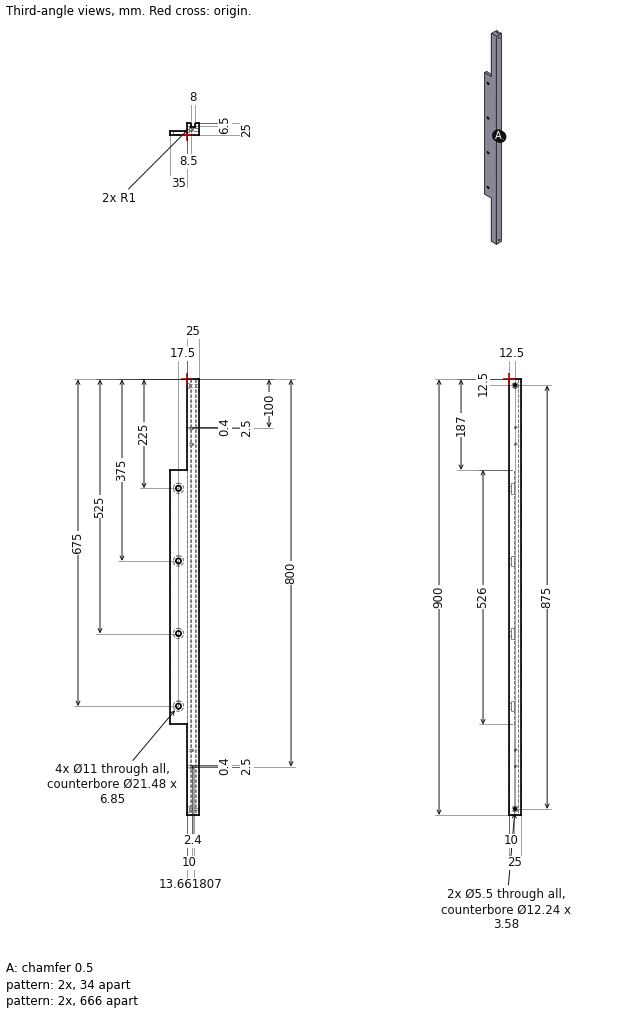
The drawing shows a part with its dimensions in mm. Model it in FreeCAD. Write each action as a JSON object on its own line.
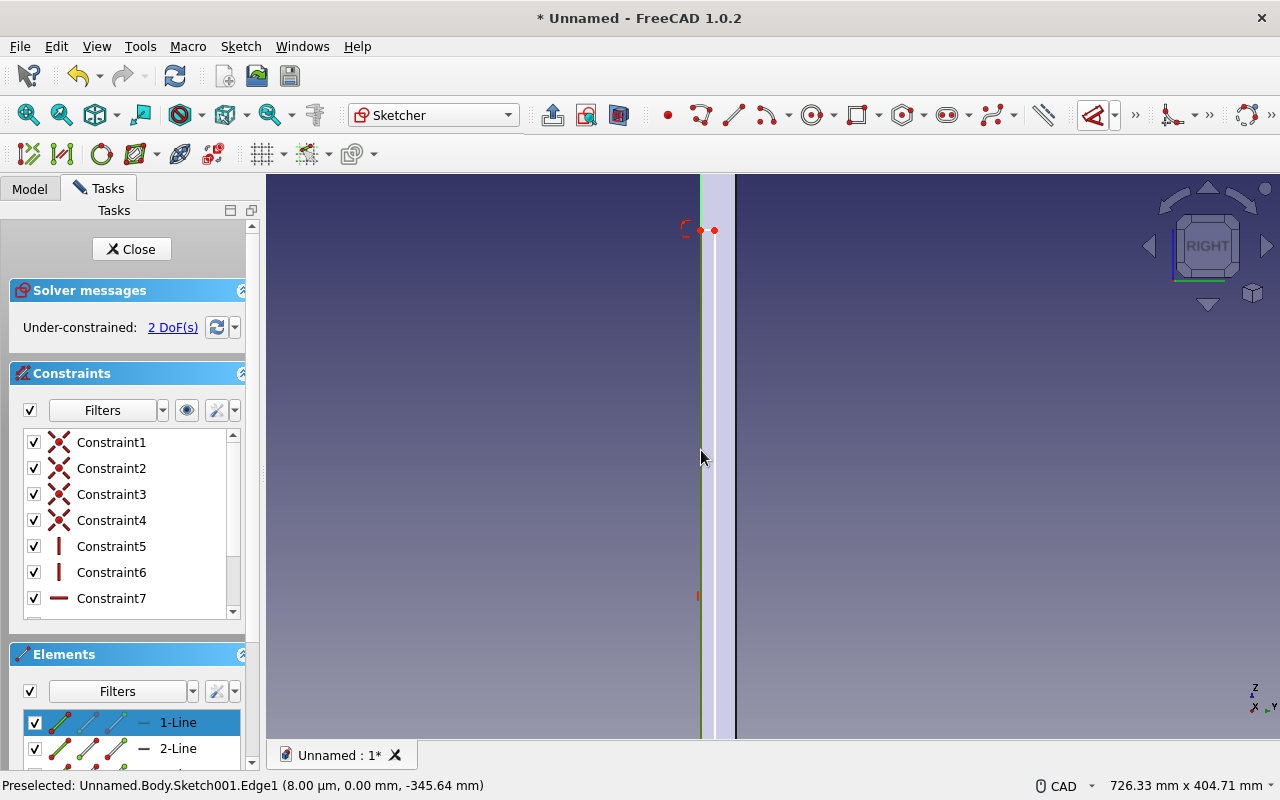
{"action": "key", "text": "i"}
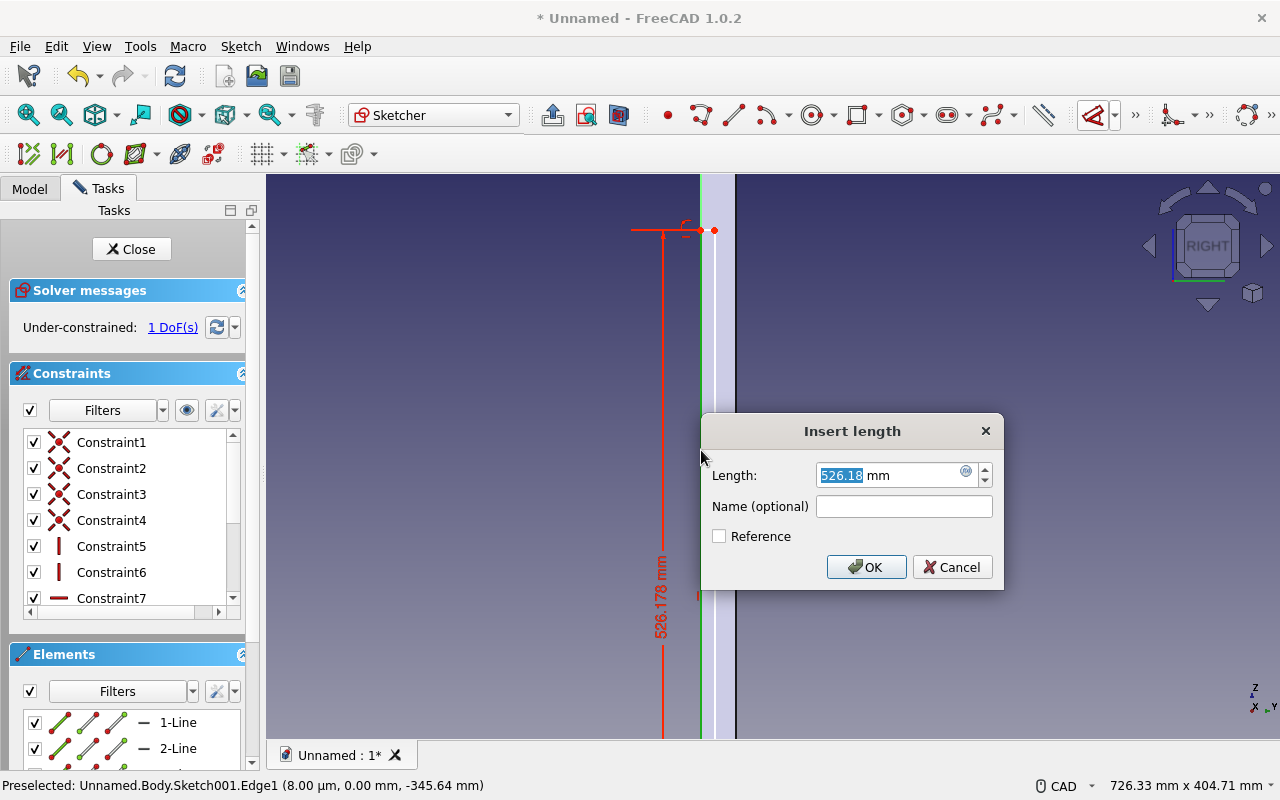
{"action": "type", "text": "526"}
{"action": "key", "text": "Return"}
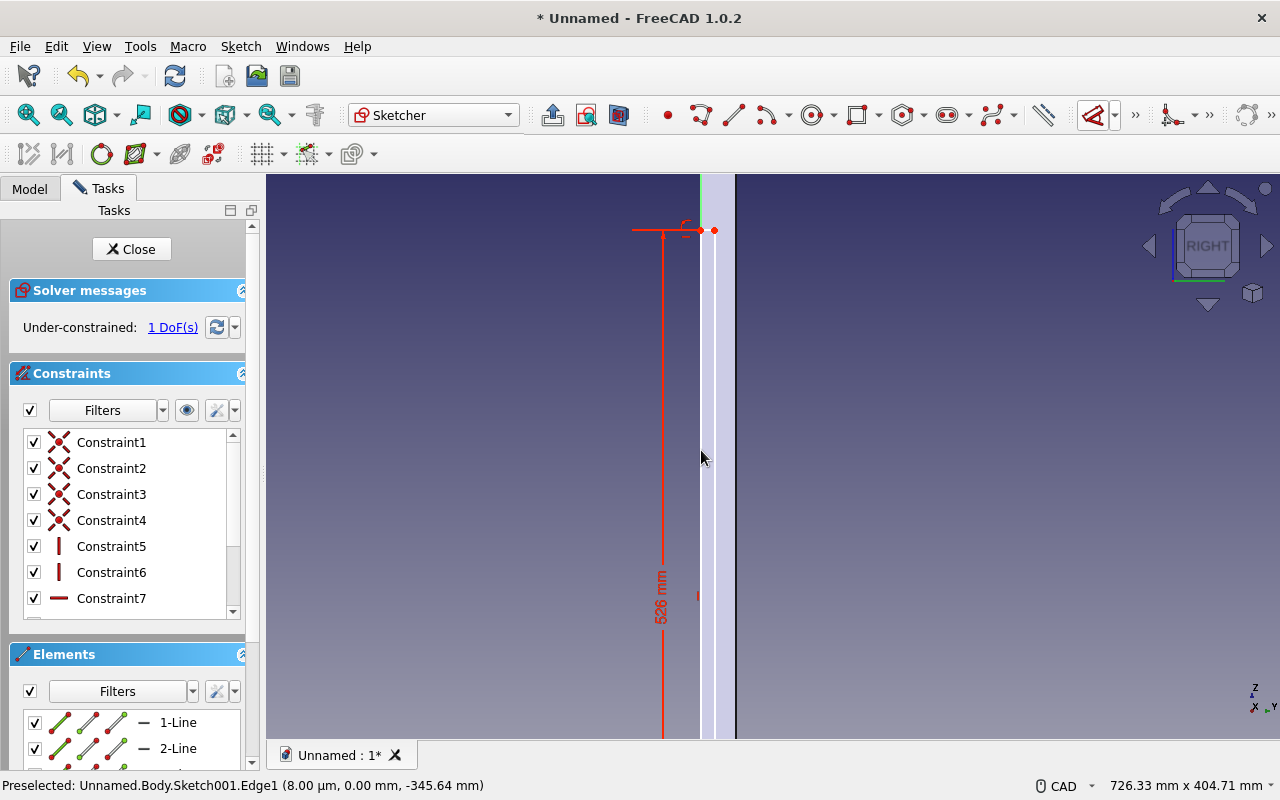
{"action": "left_click", "coordinate": [701, 230]}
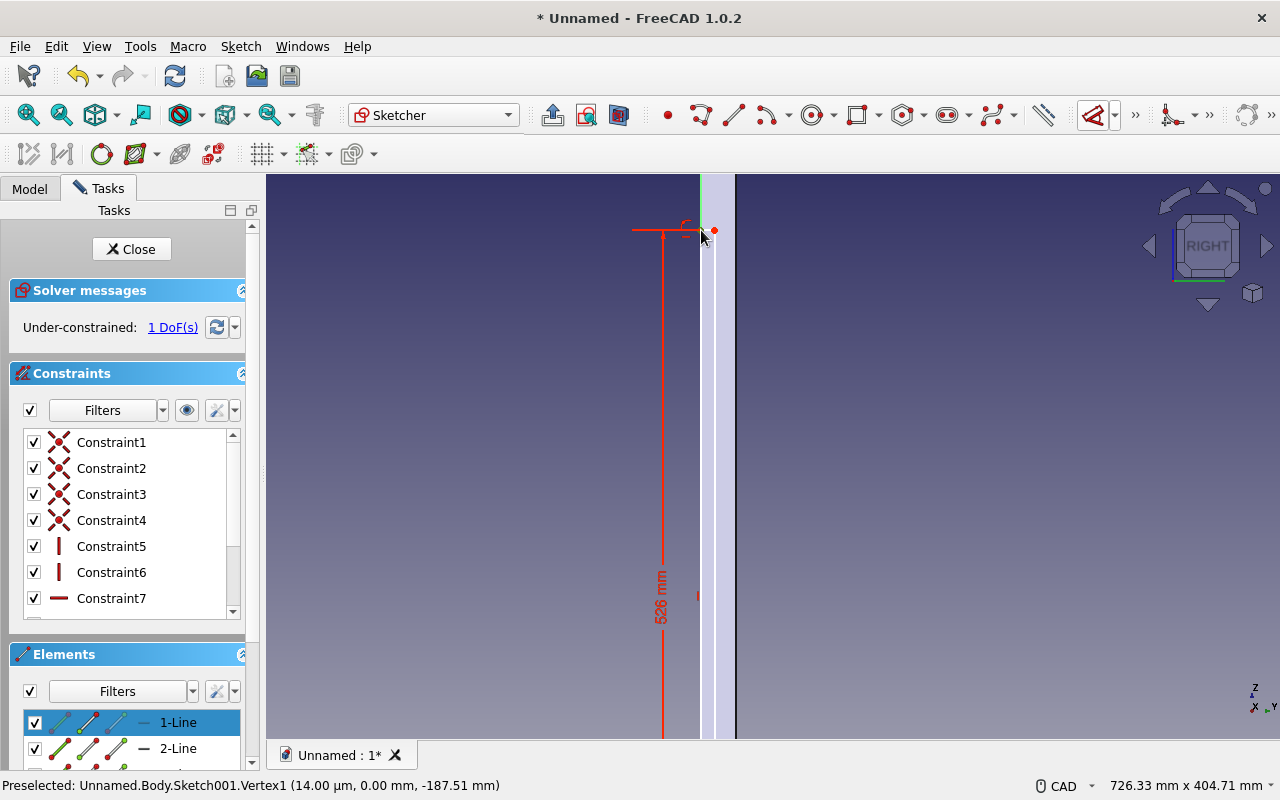
{"action": "key", "text": "i"}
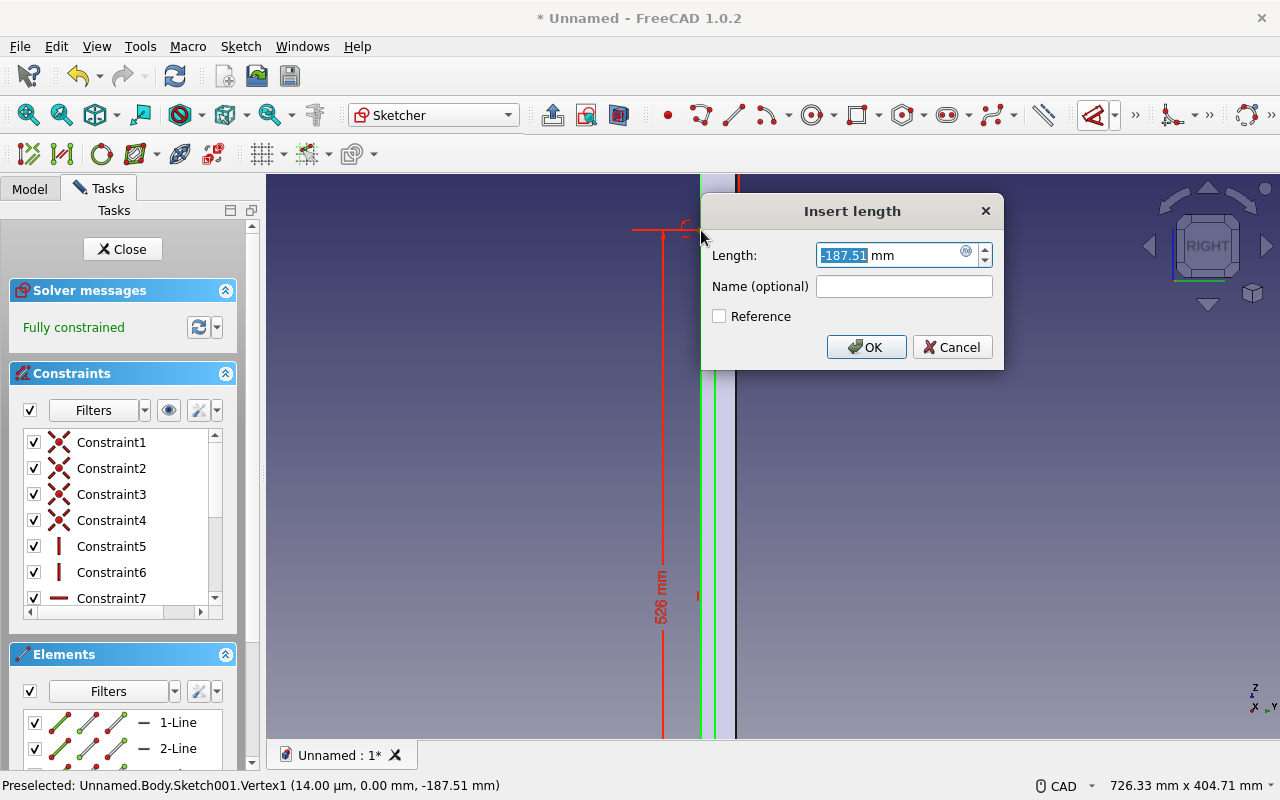
{"action": "type", "text": "-187"}
{"action": "key", "text": "Return"}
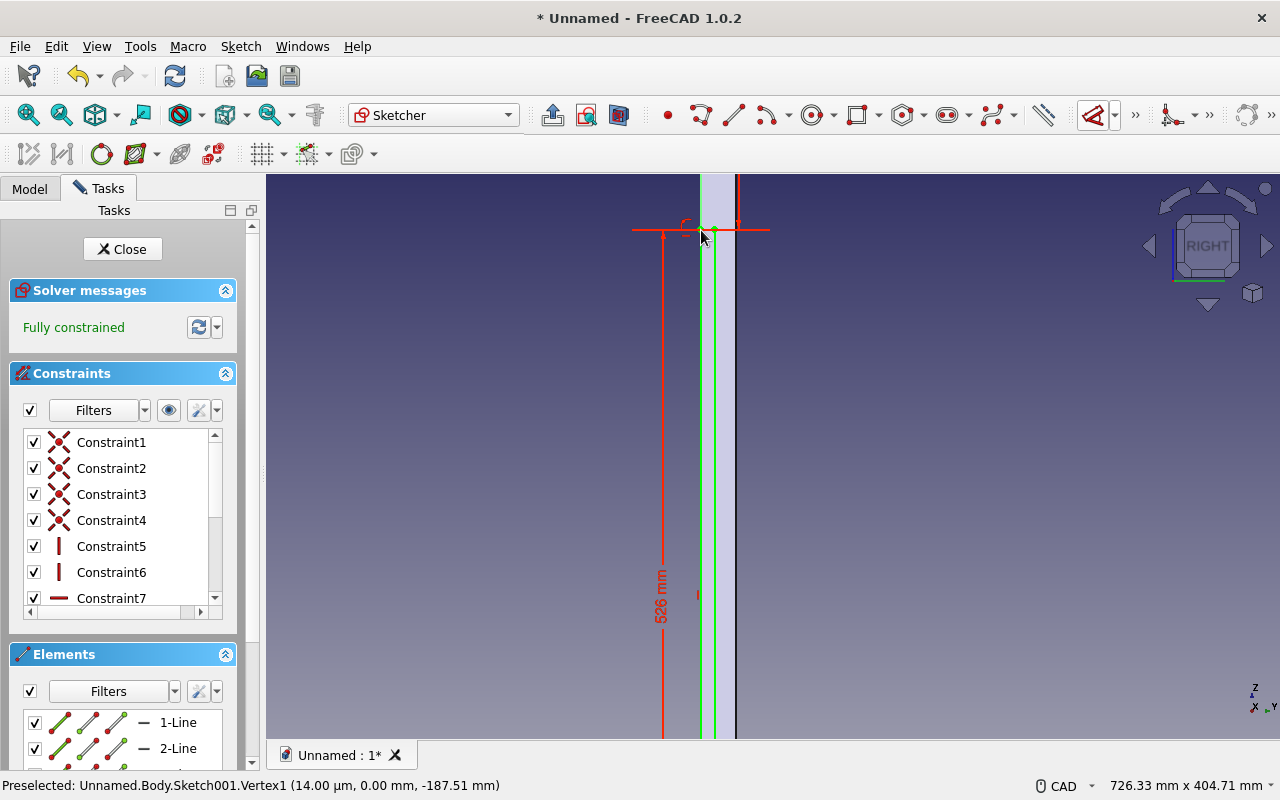
{"action": "left_click", "coordinate": [123, 249]}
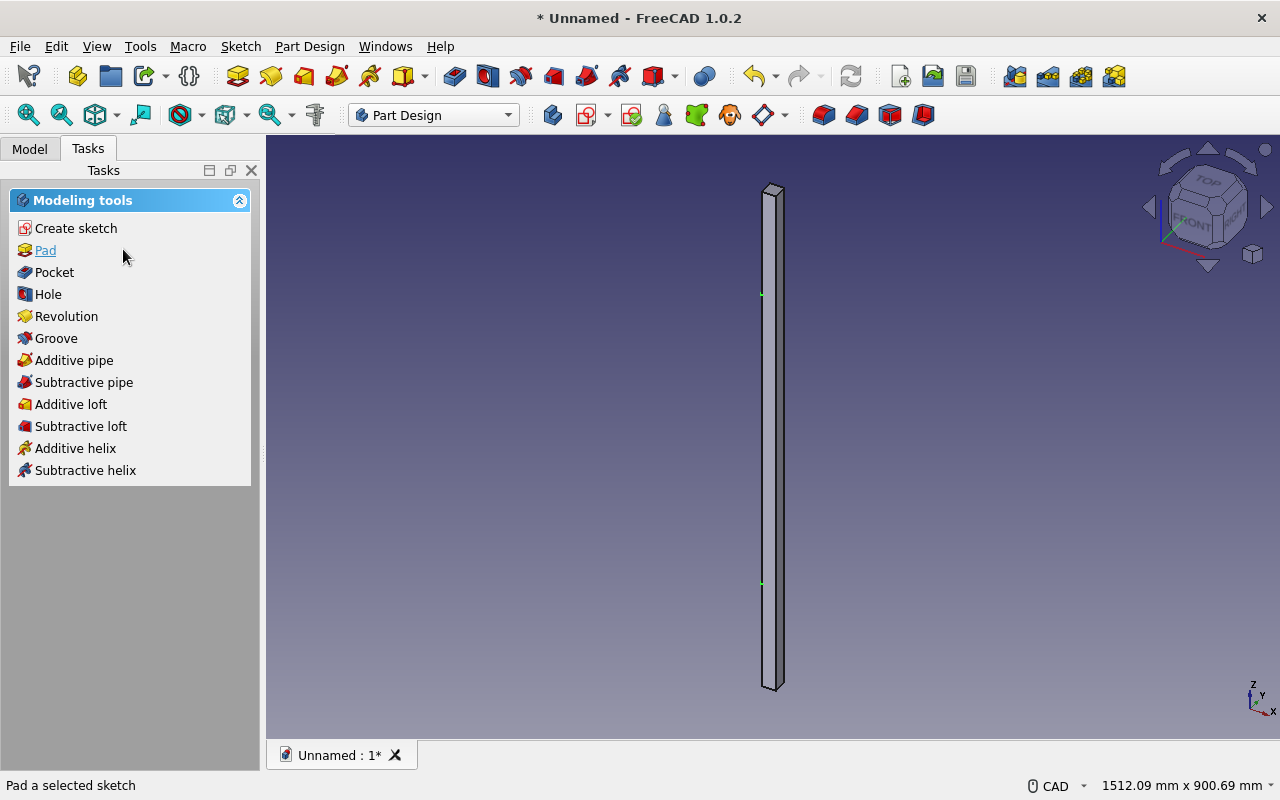
{"action": "left_click", "coordinate": [238, 76]}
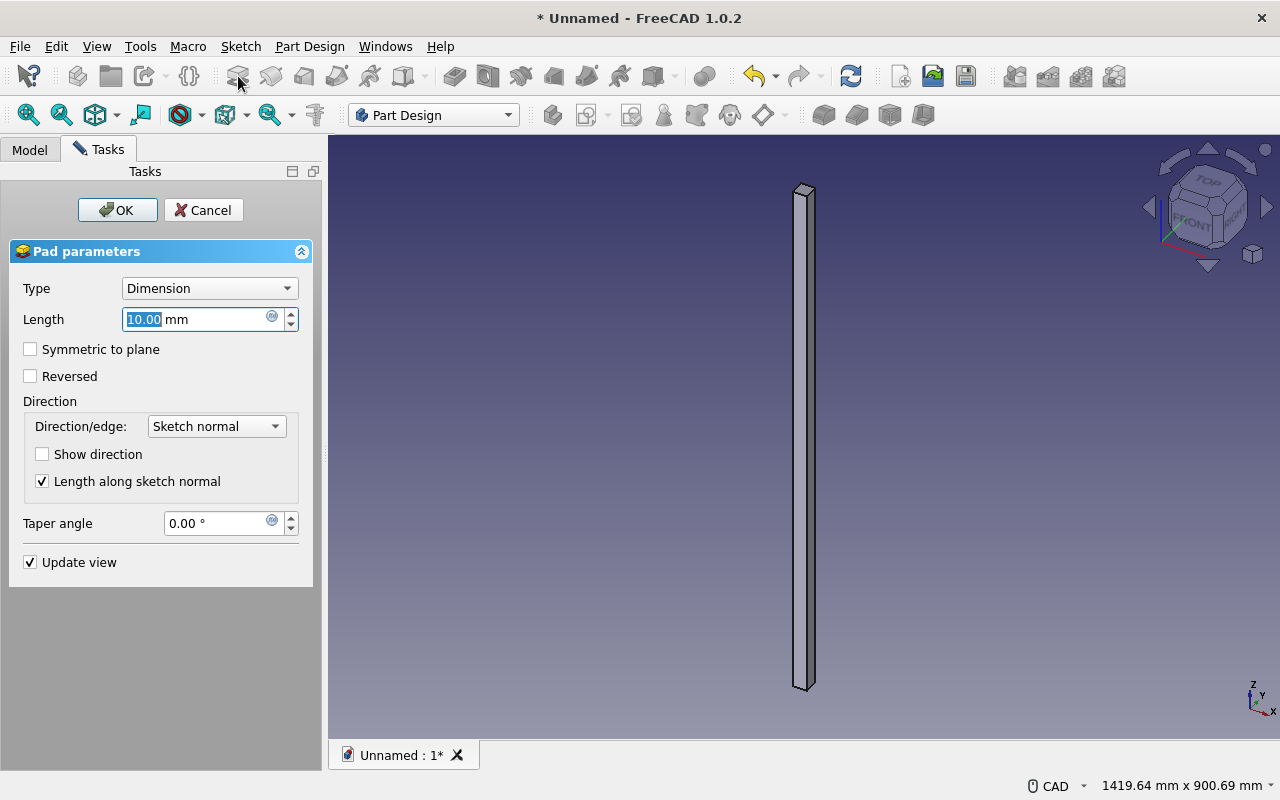
{"action": "type", "text": "35"}
{"action": "key", "text": "Tab"}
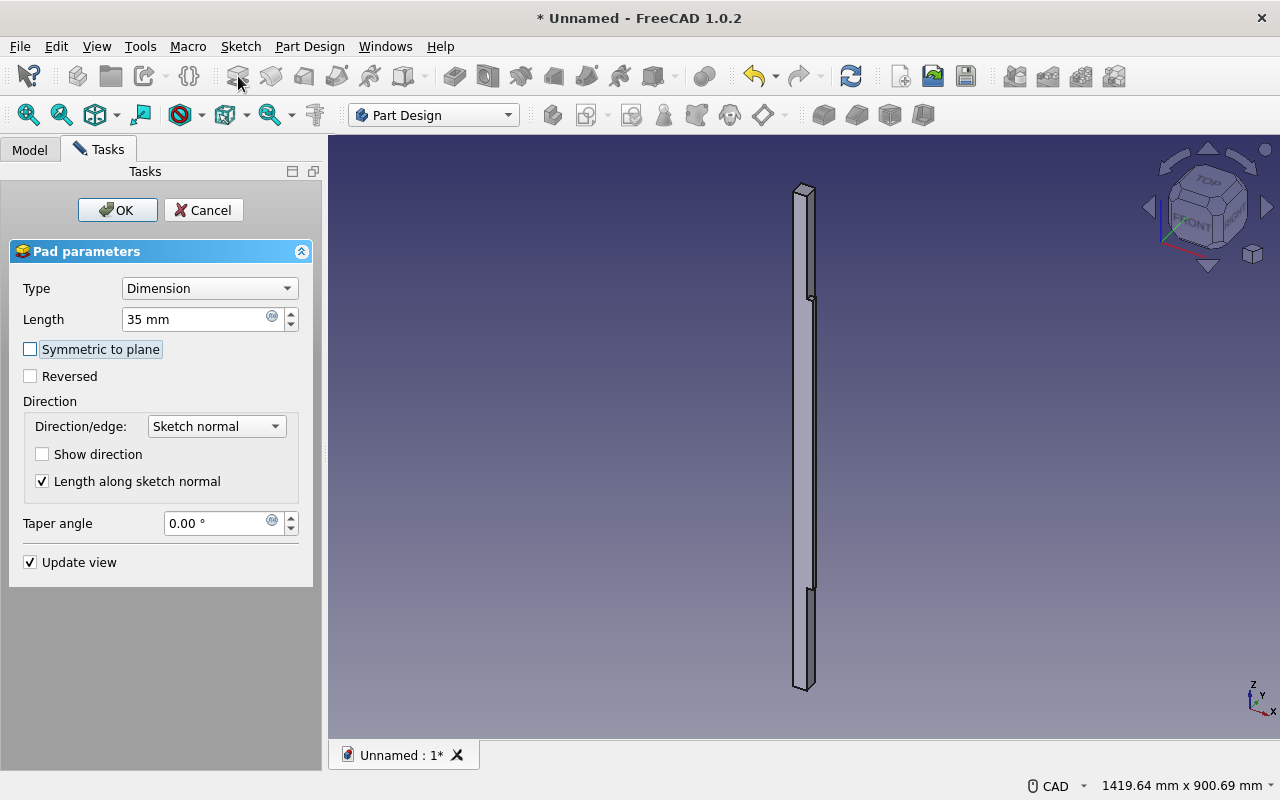
{"action": "left_click", "coordinate": [31, 376]}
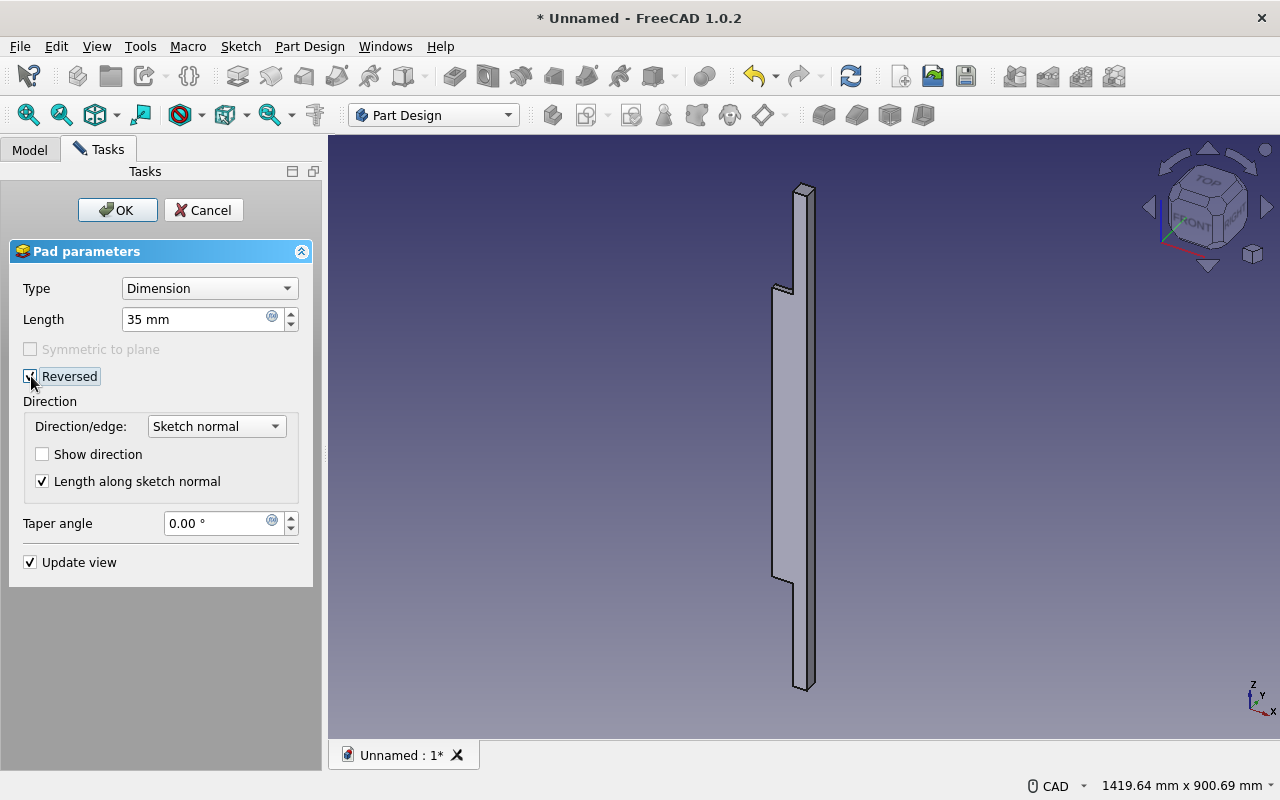
{"action": "left_click", "coordinate": [118, 210]}